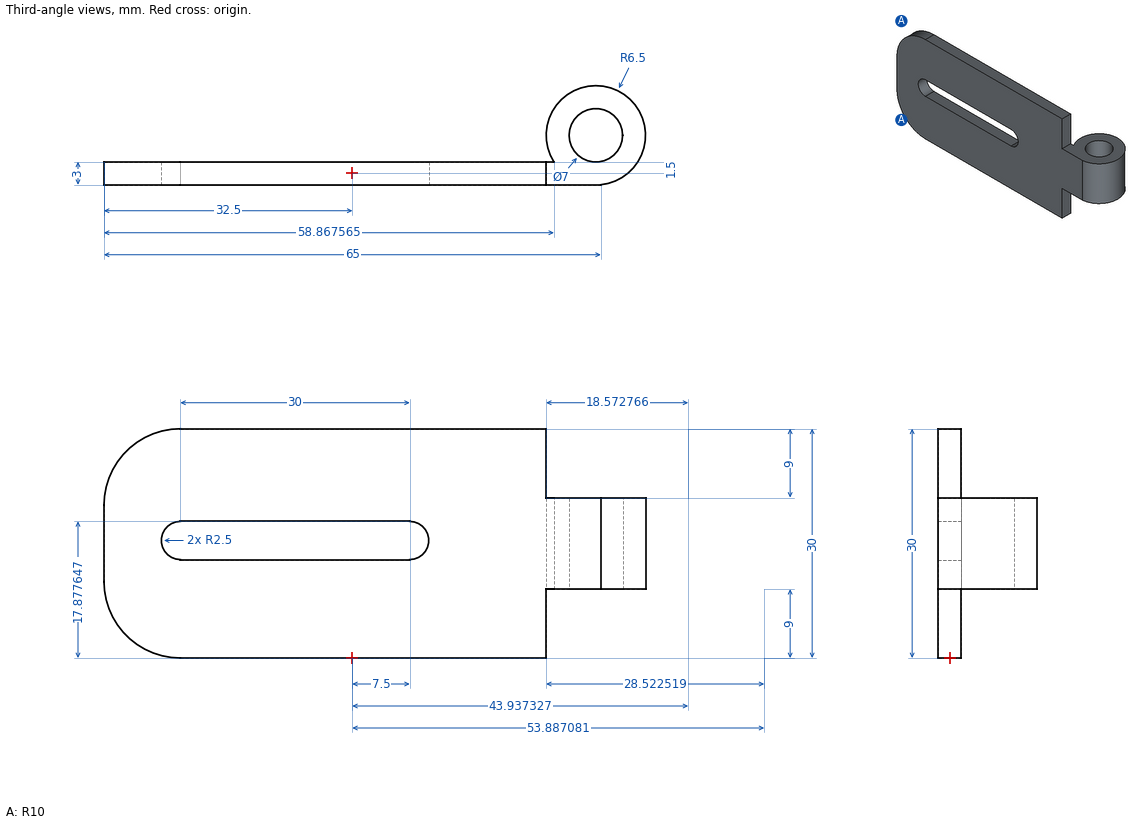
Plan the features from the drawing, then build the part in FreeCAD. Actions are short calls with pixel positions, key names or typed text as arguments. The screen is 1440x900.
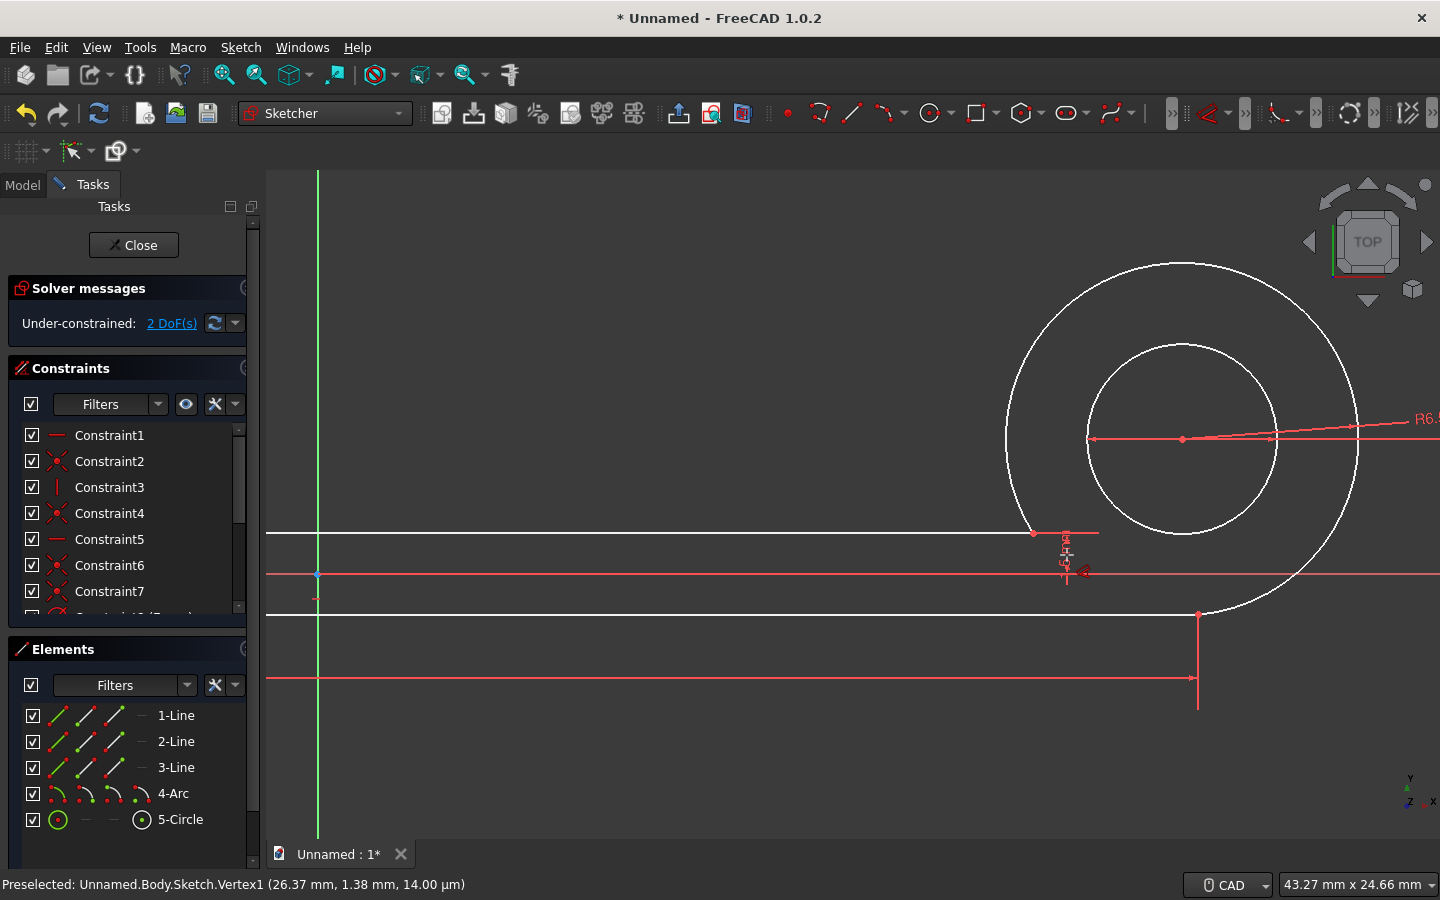
scroll(1033, 537, down, 5)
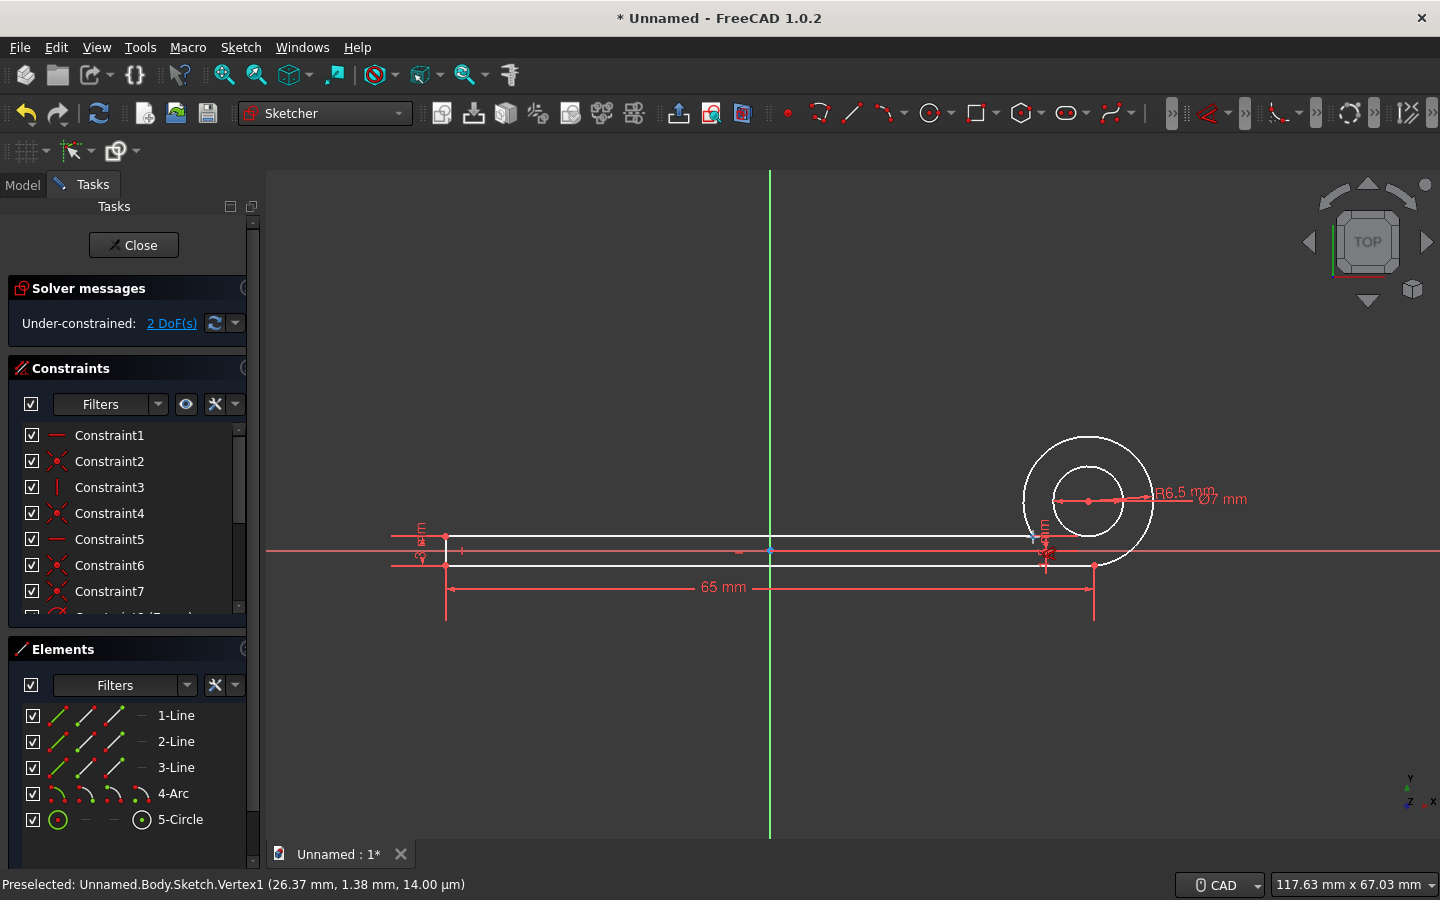
click(446, 536)
click(608, 585)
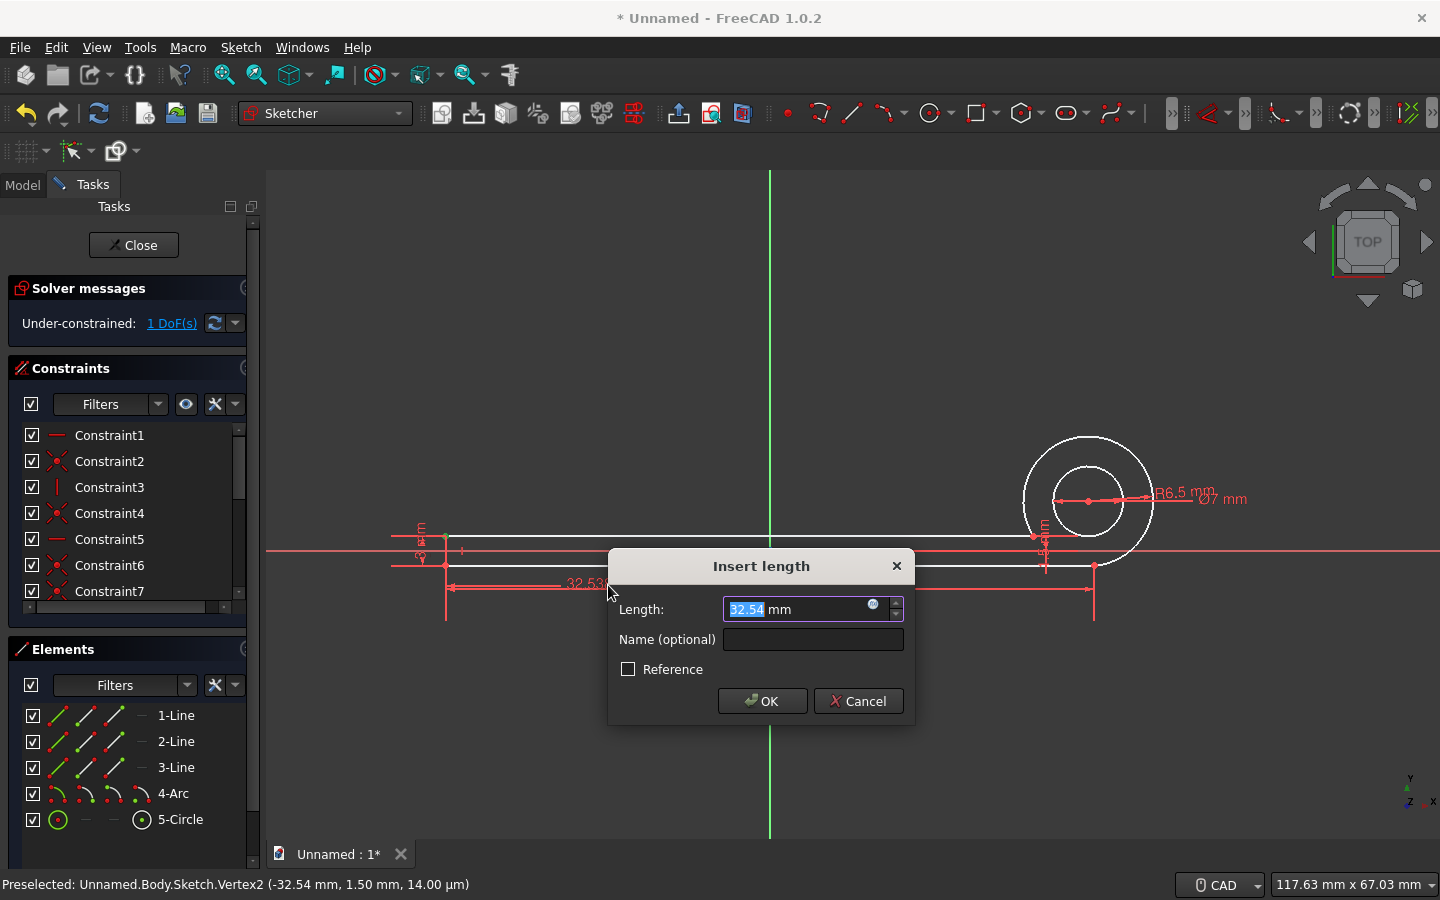
text(32.5)
key(Return)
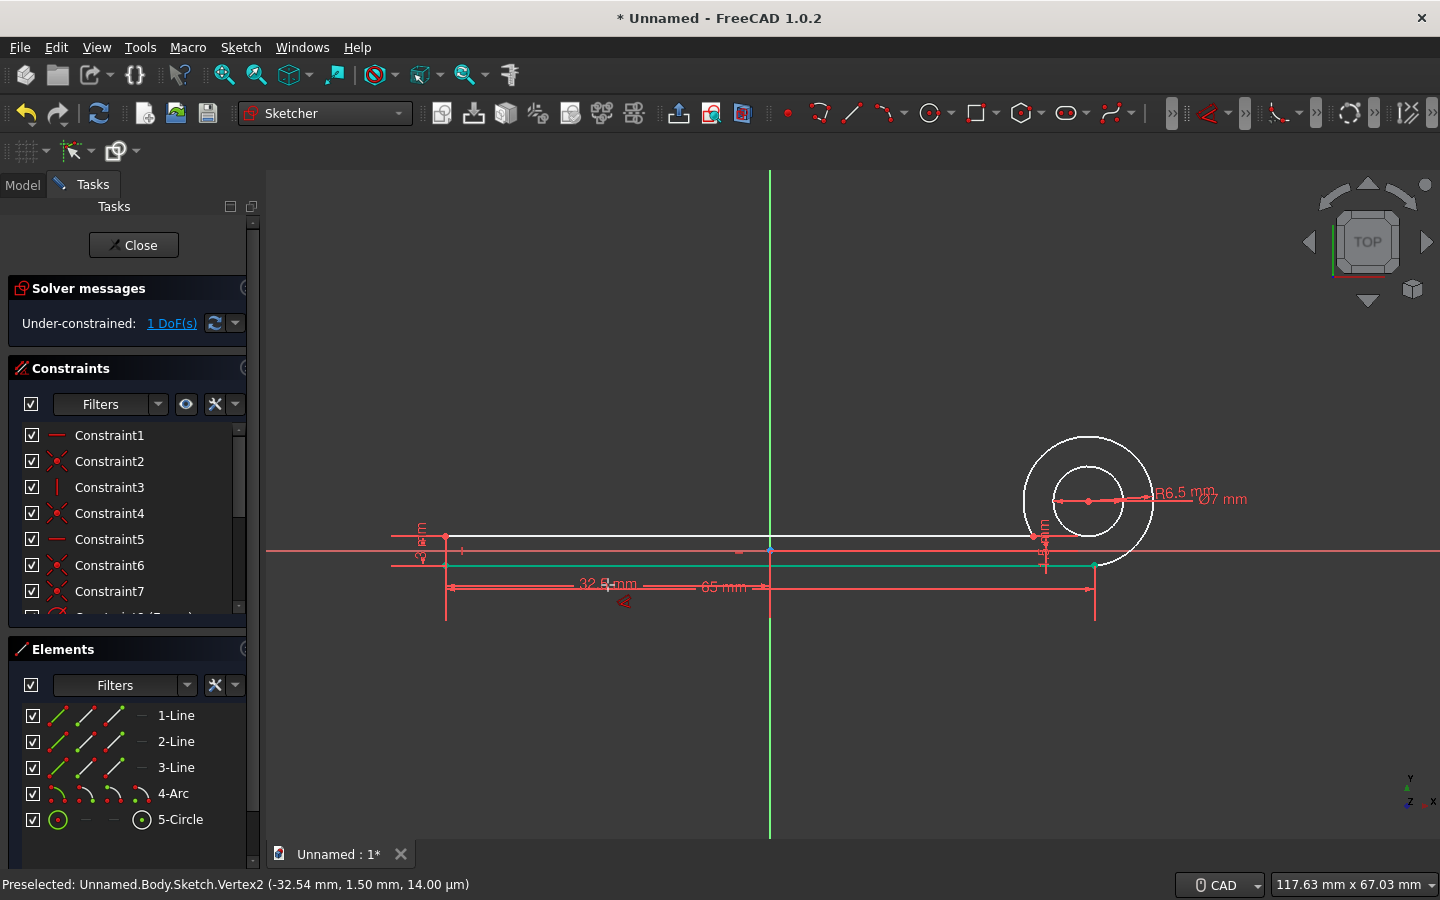
click(857, 536)
click(740, 502)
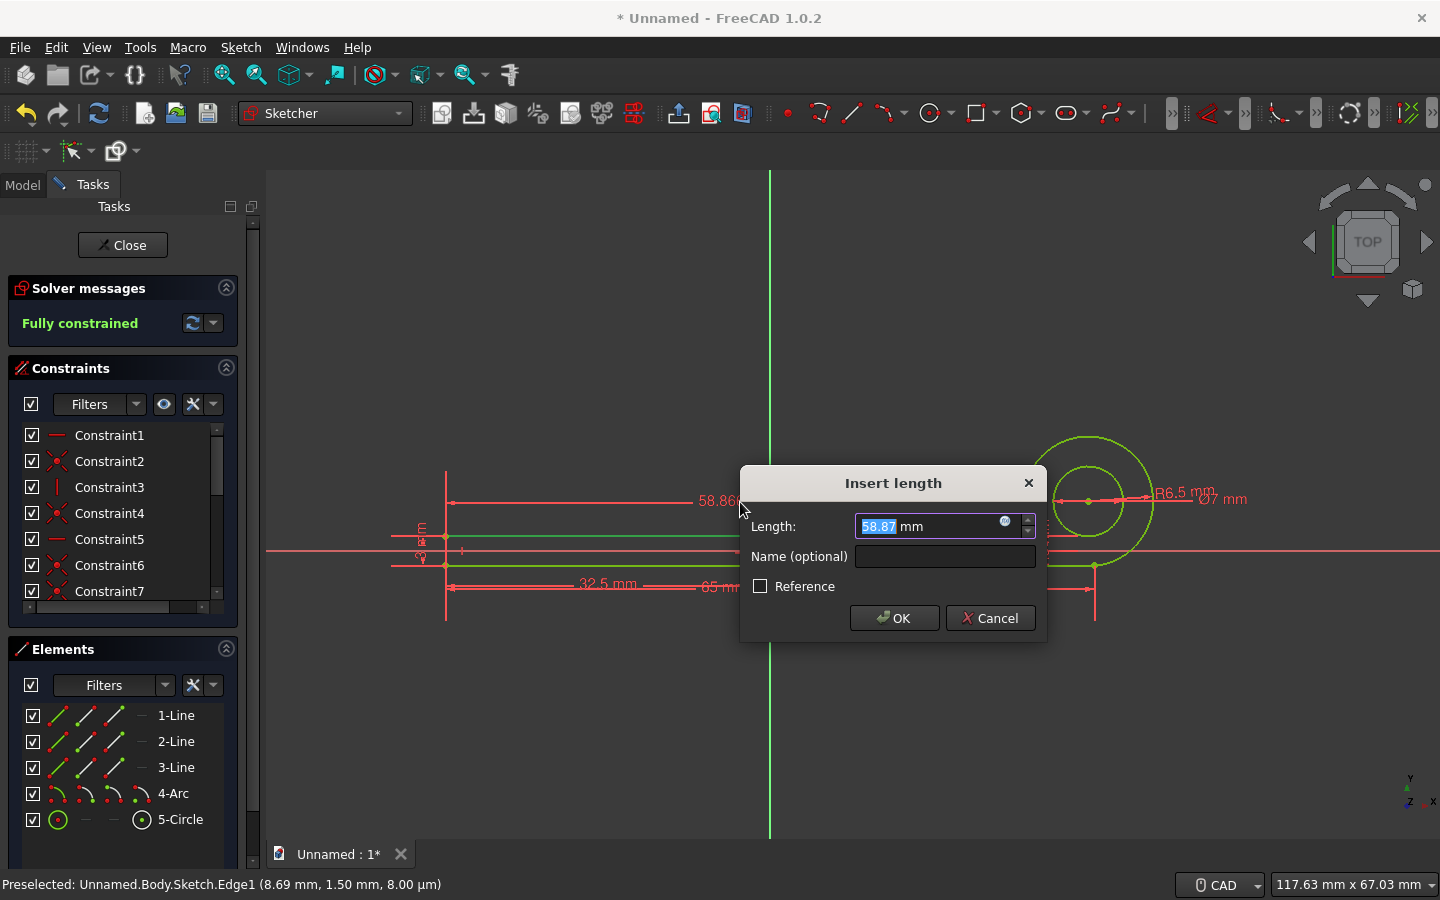
text(58.867565)
key(Return)
key(Escape)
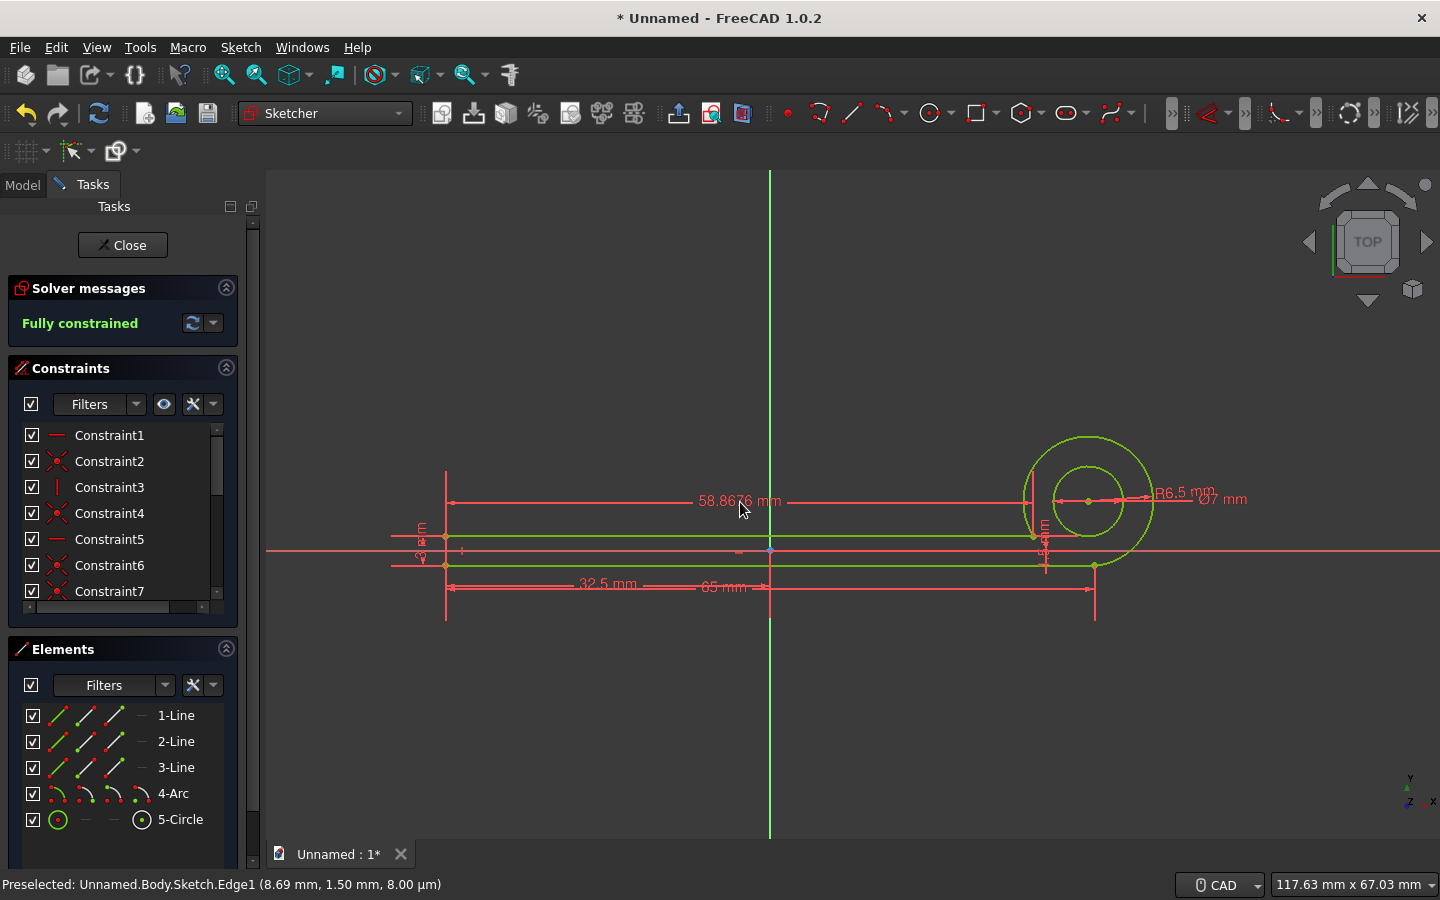
click(123, 245)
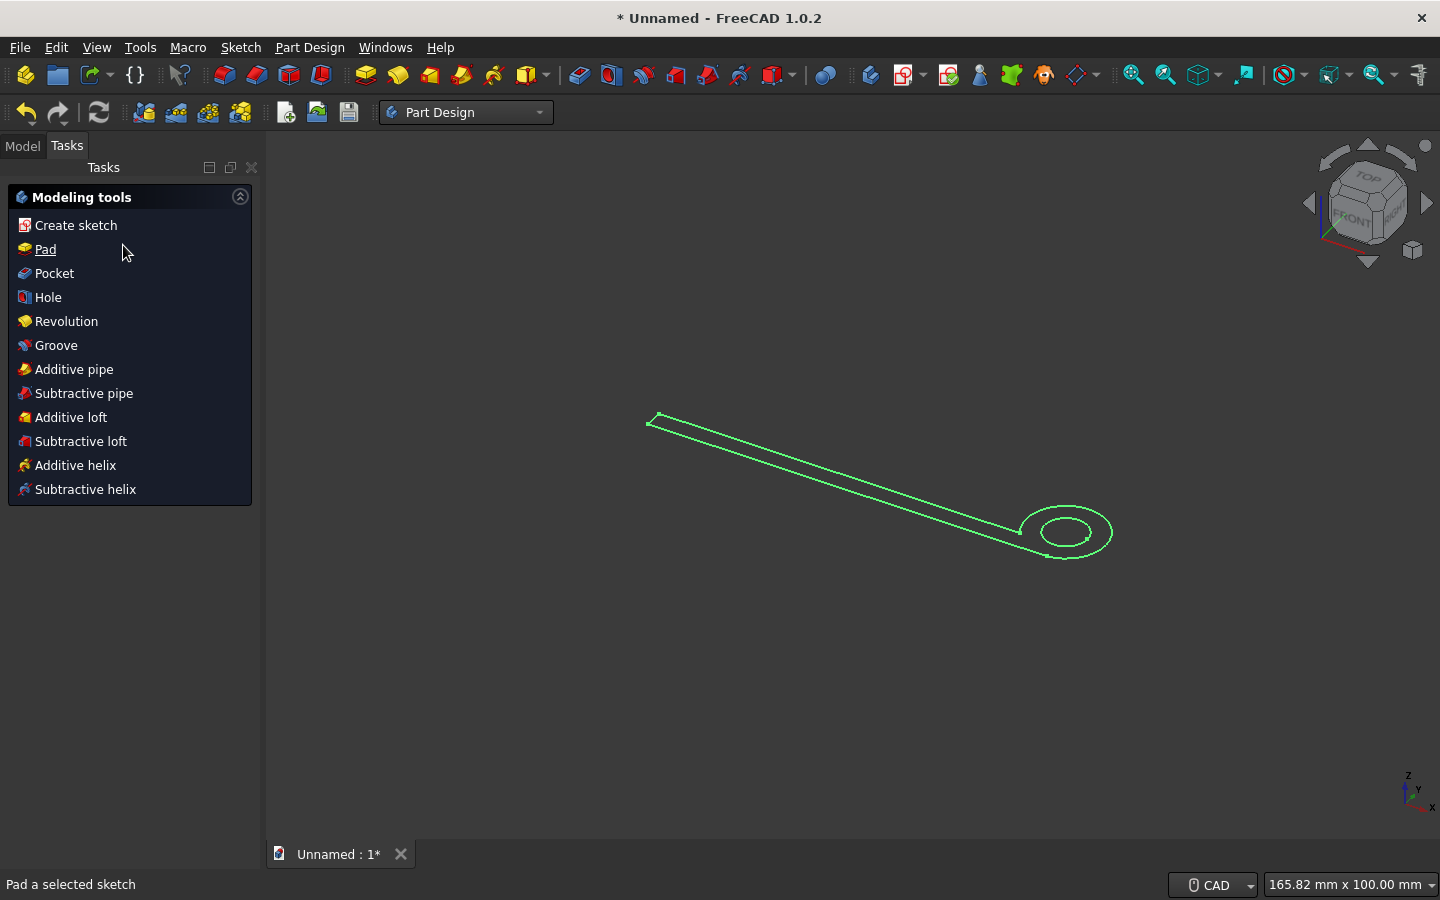
click(366, 76)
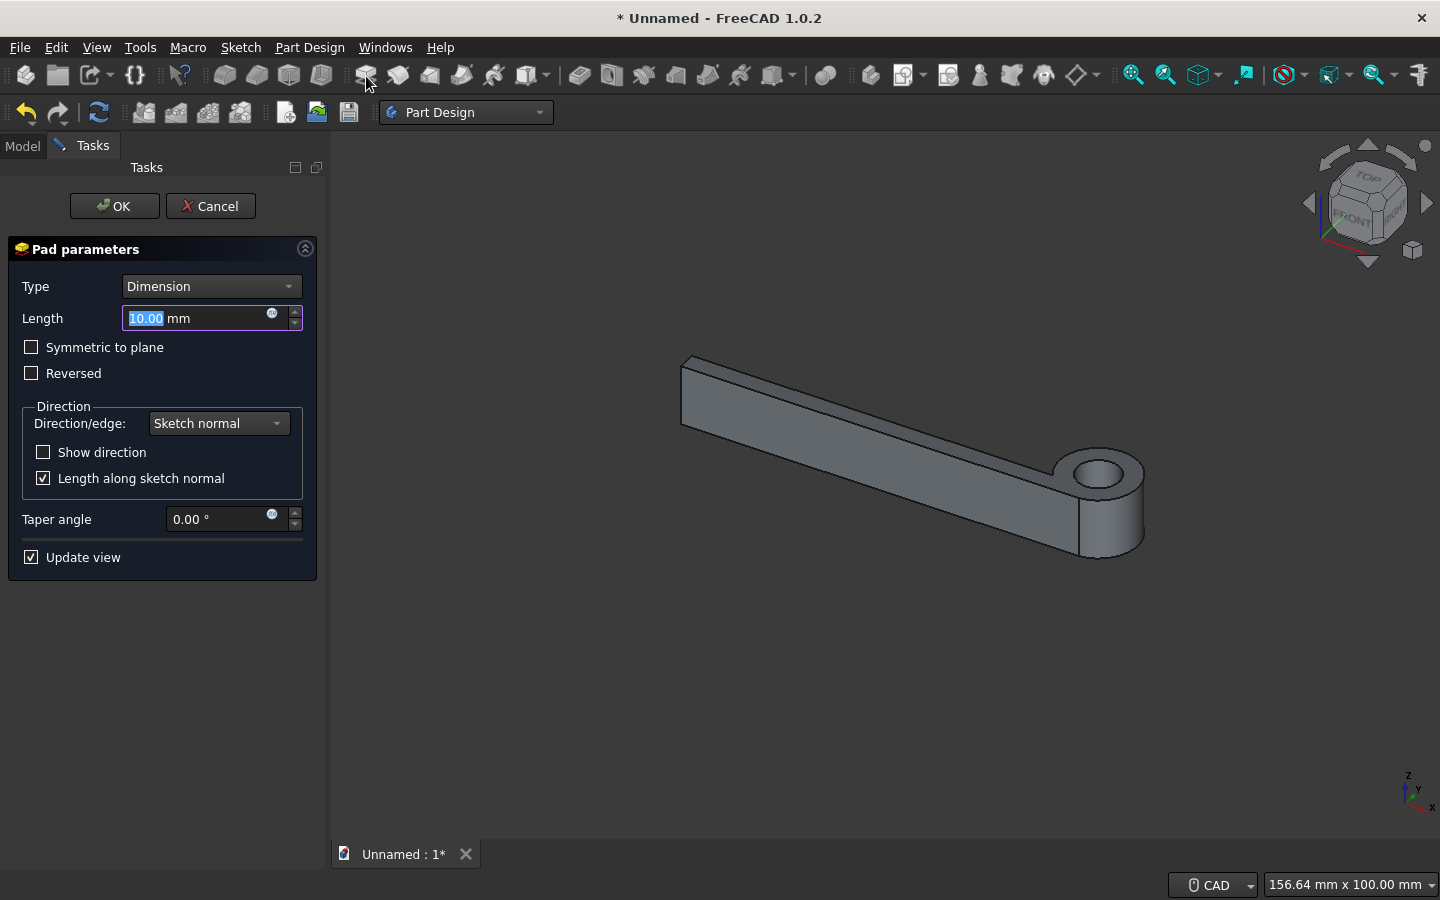
text(30)
key(Tab)